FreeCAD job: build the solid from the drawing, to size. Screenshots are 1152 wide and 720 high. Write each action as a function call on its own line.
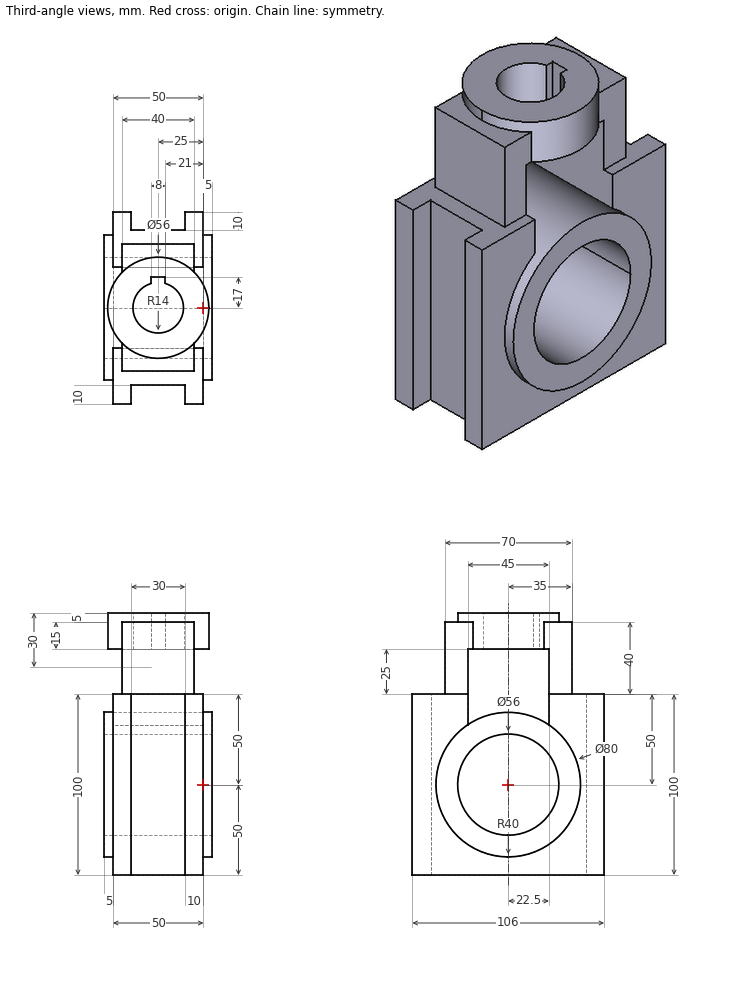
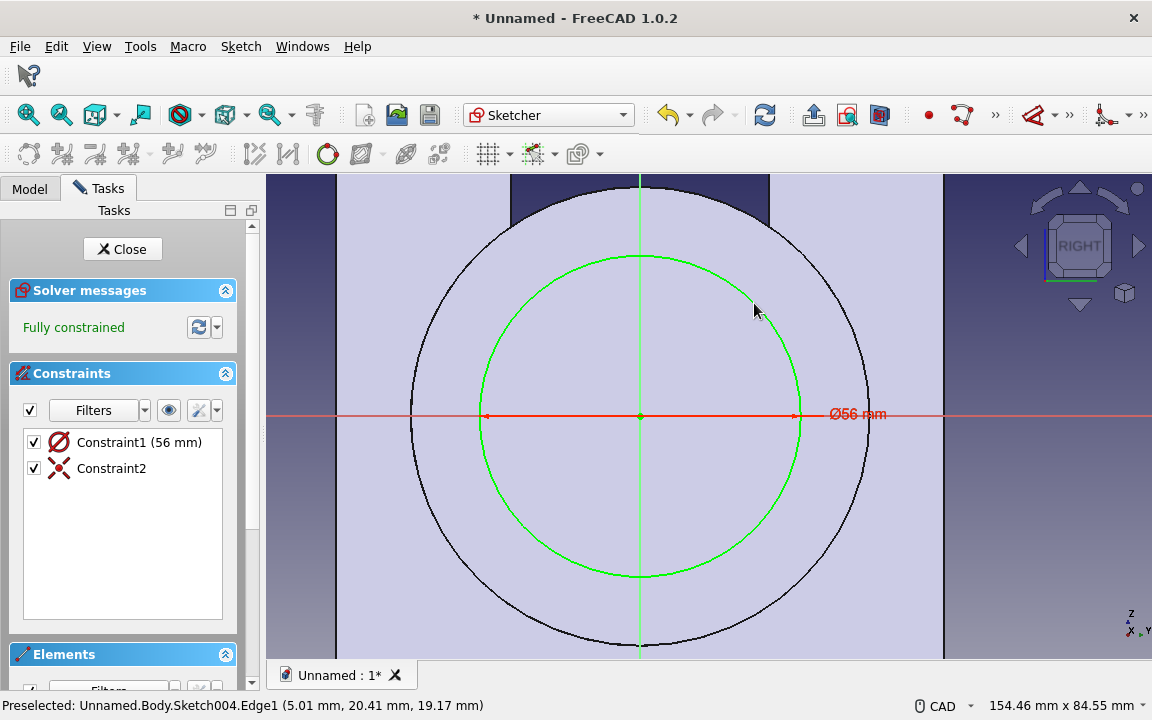
click(123, 249)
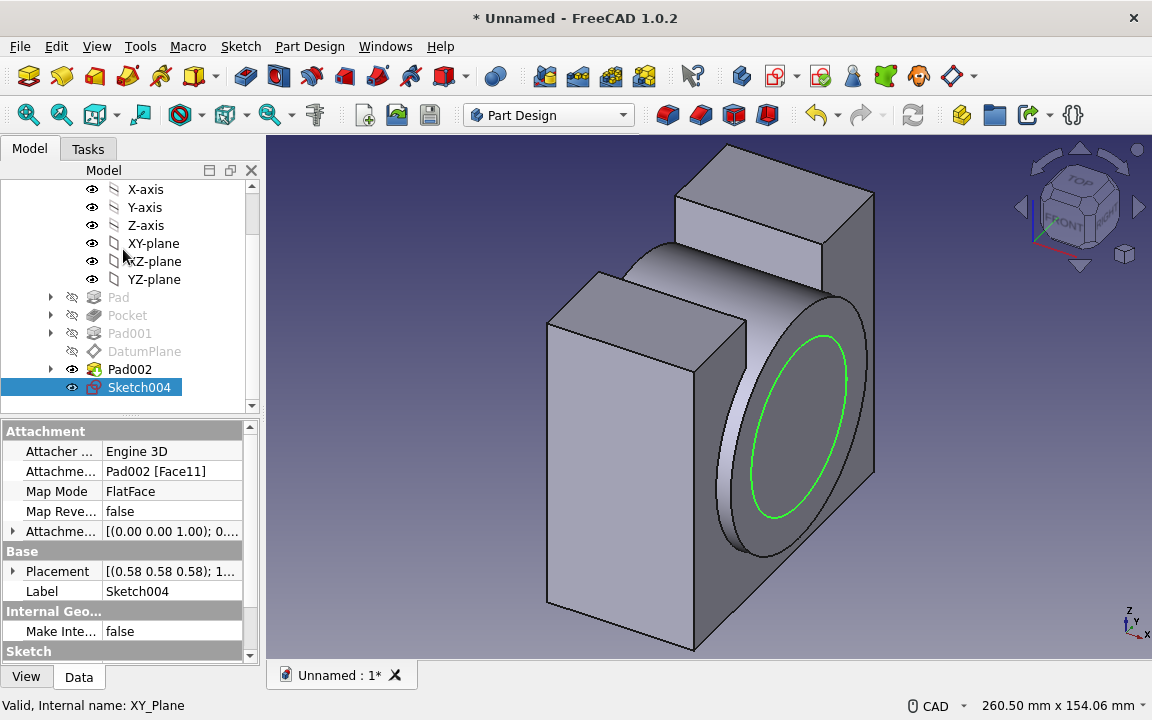
click(246, 76)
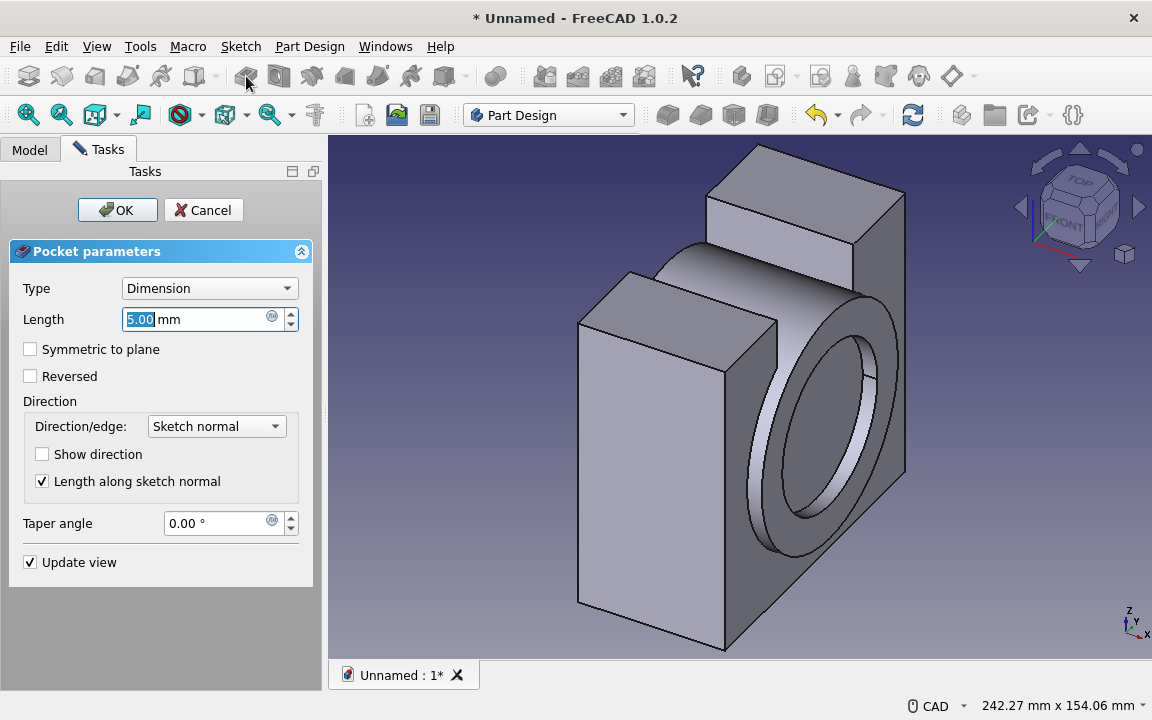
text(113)
key(Tab)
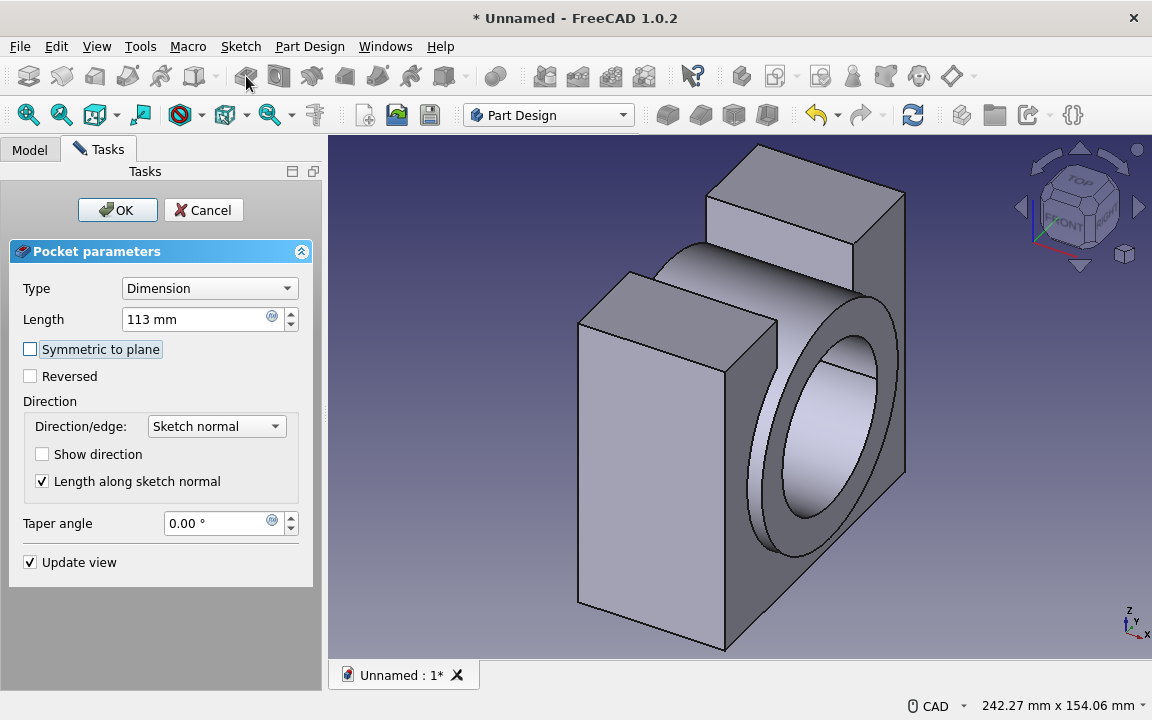
click(118, 210)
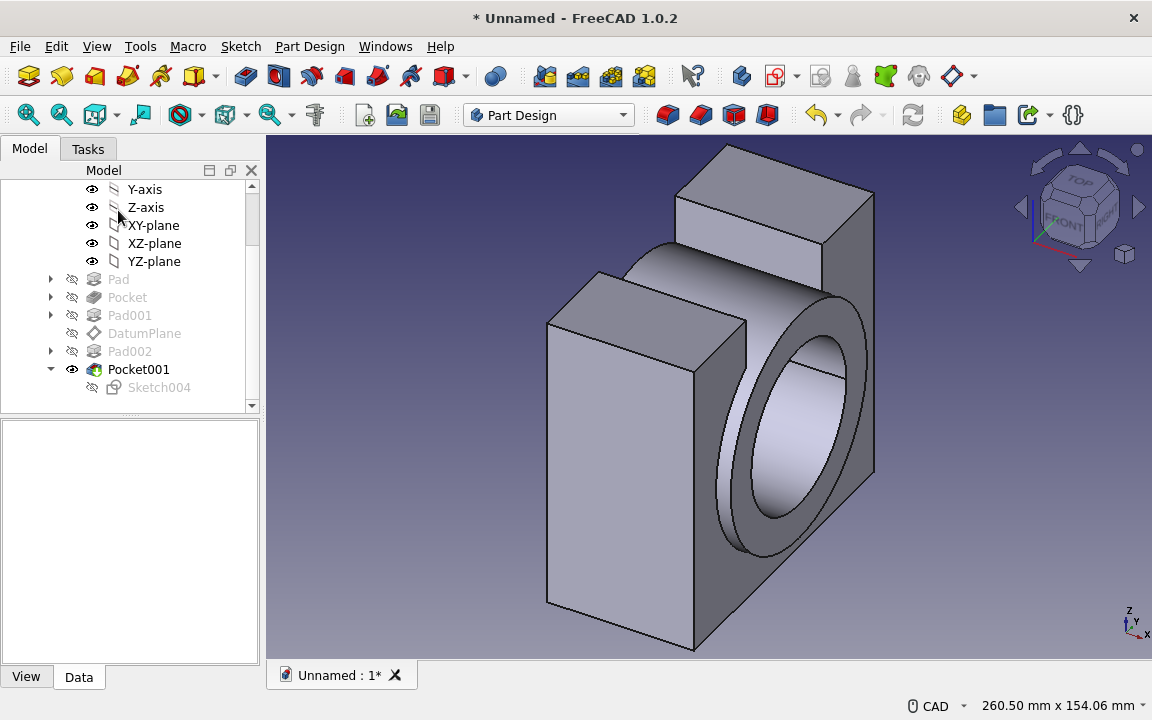
key(4)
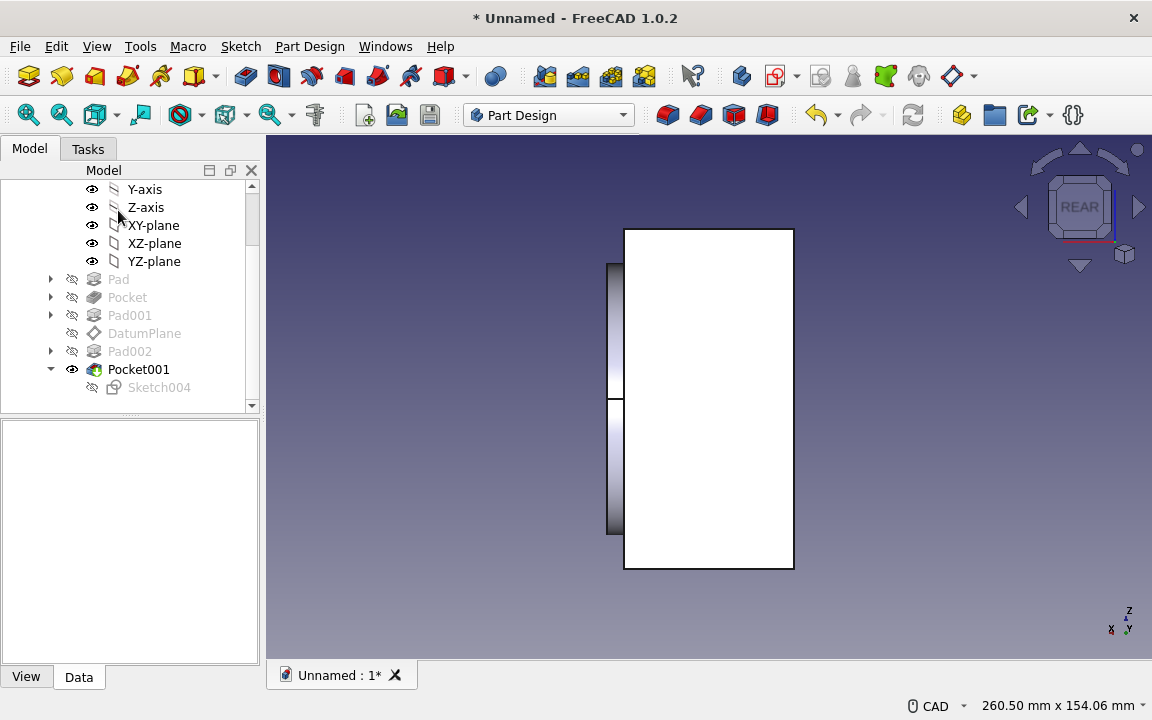
click(709, 398)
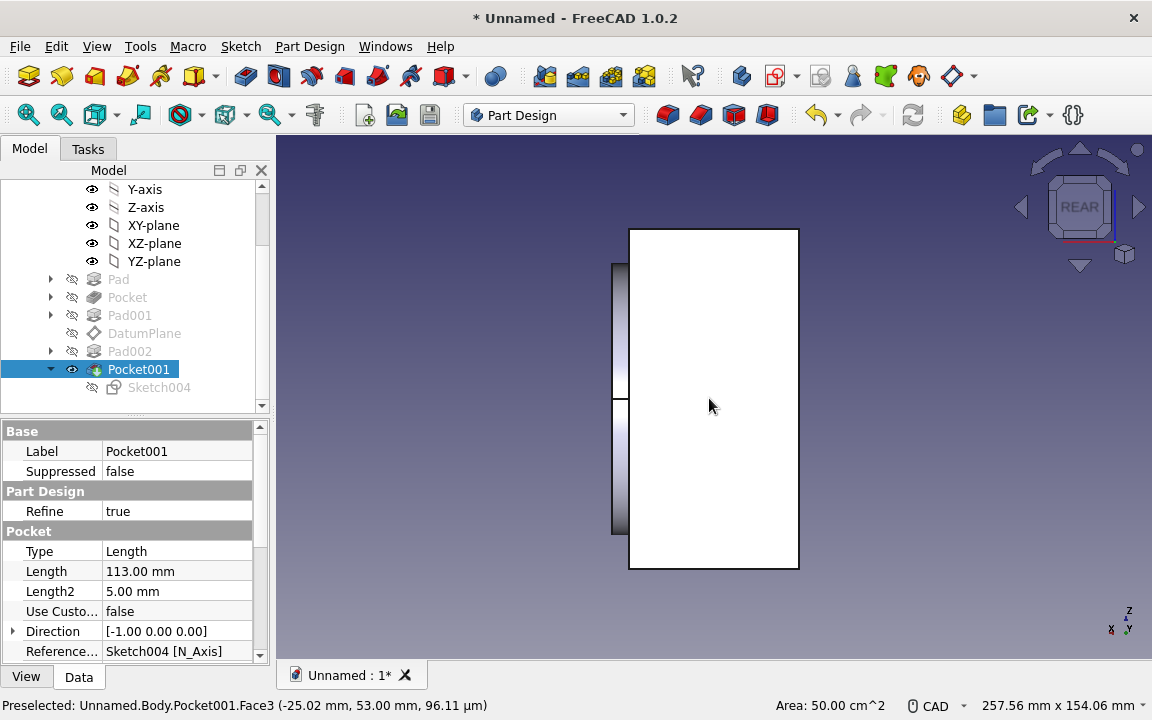
click(774, 76)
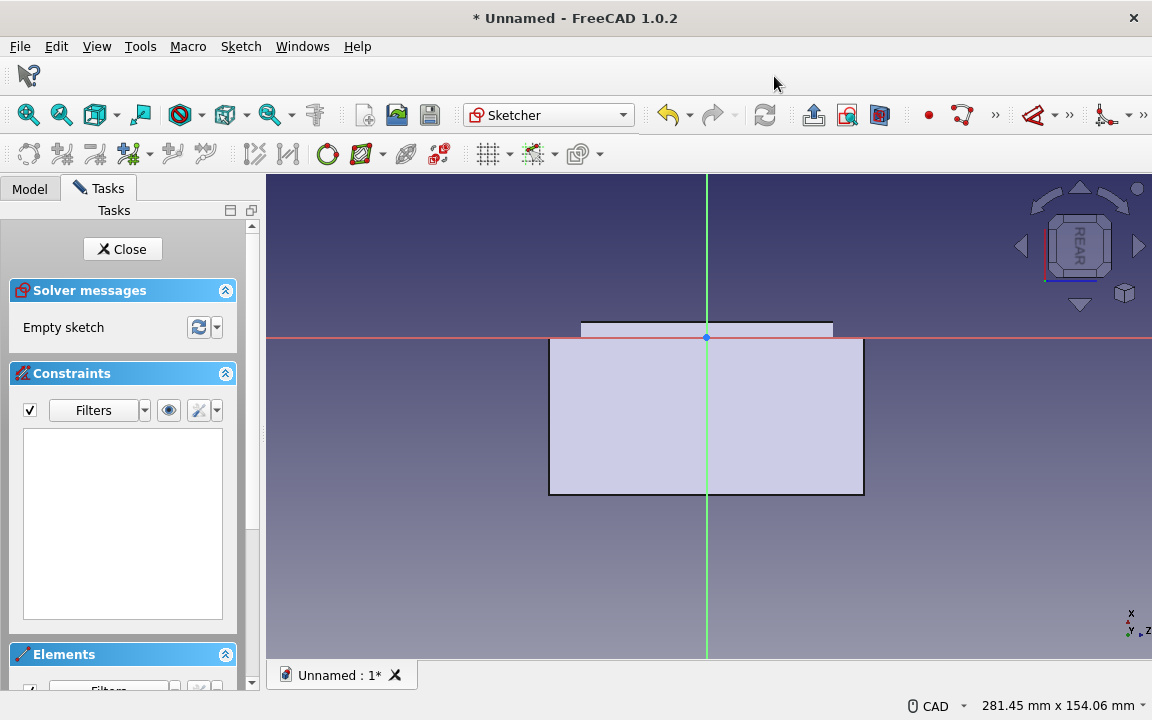
scroll(842, 369, up, 2)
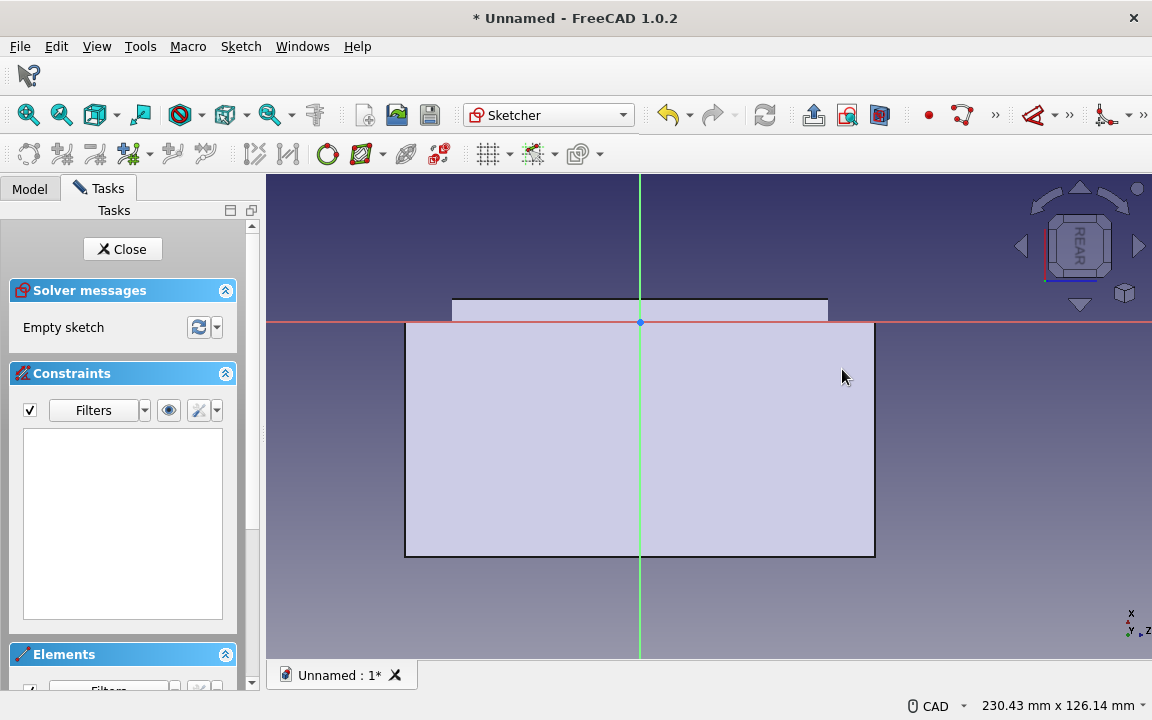
key(g)
key(r)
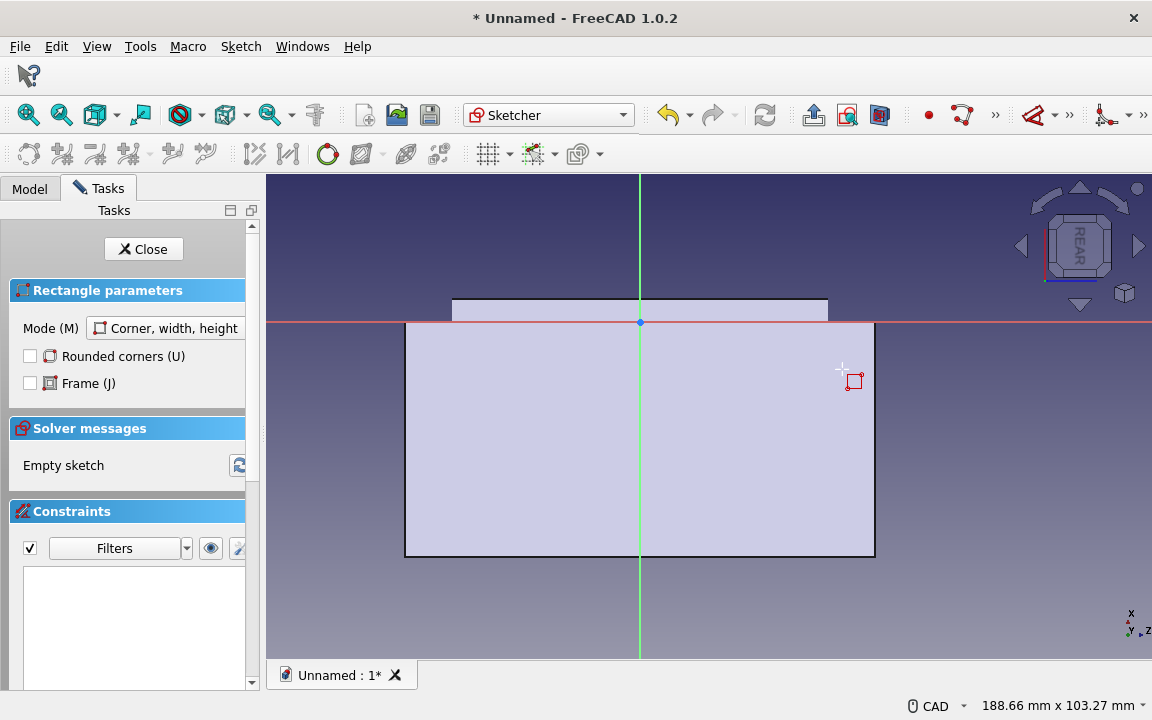
click(405, 369)
move(875, 510)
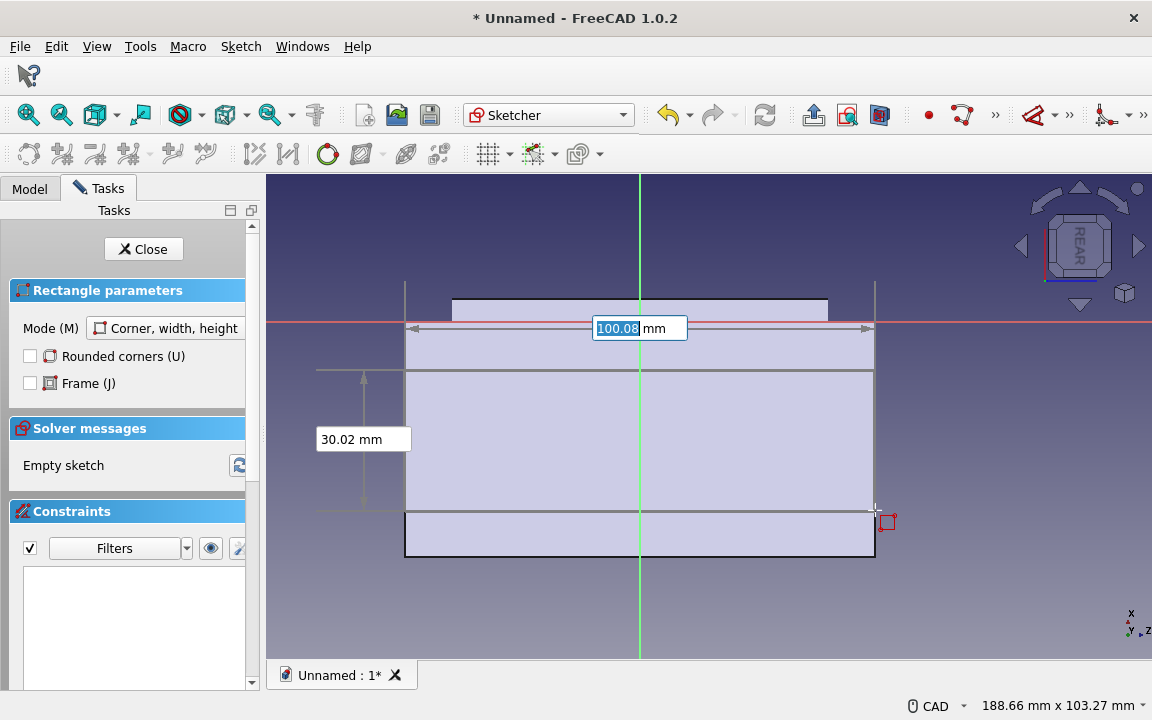
text(100)
key(Tab)
text(30)
key(Return)
key(Escape)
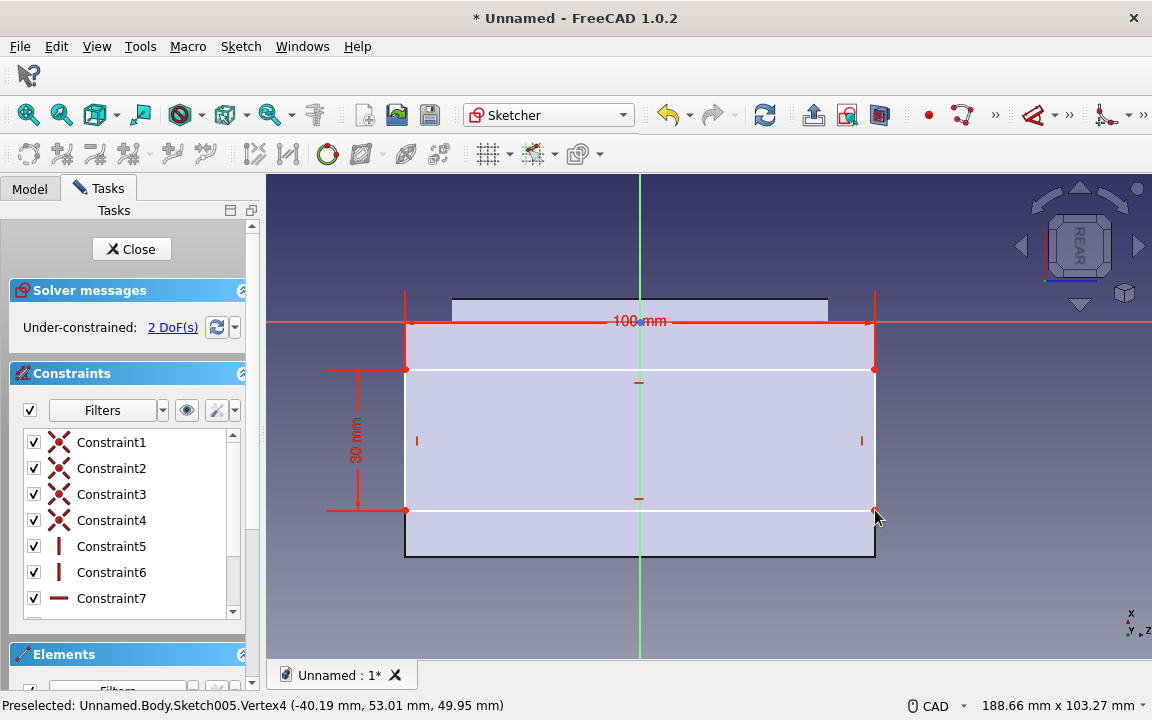
key(d)